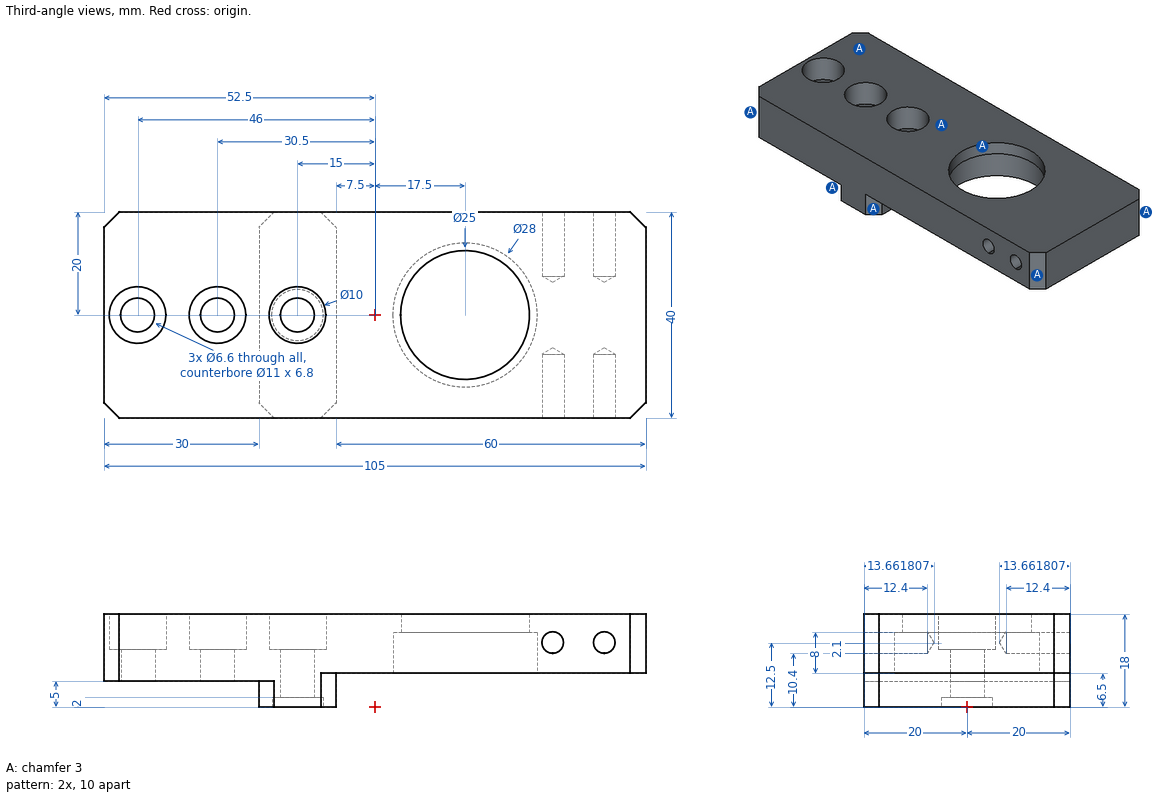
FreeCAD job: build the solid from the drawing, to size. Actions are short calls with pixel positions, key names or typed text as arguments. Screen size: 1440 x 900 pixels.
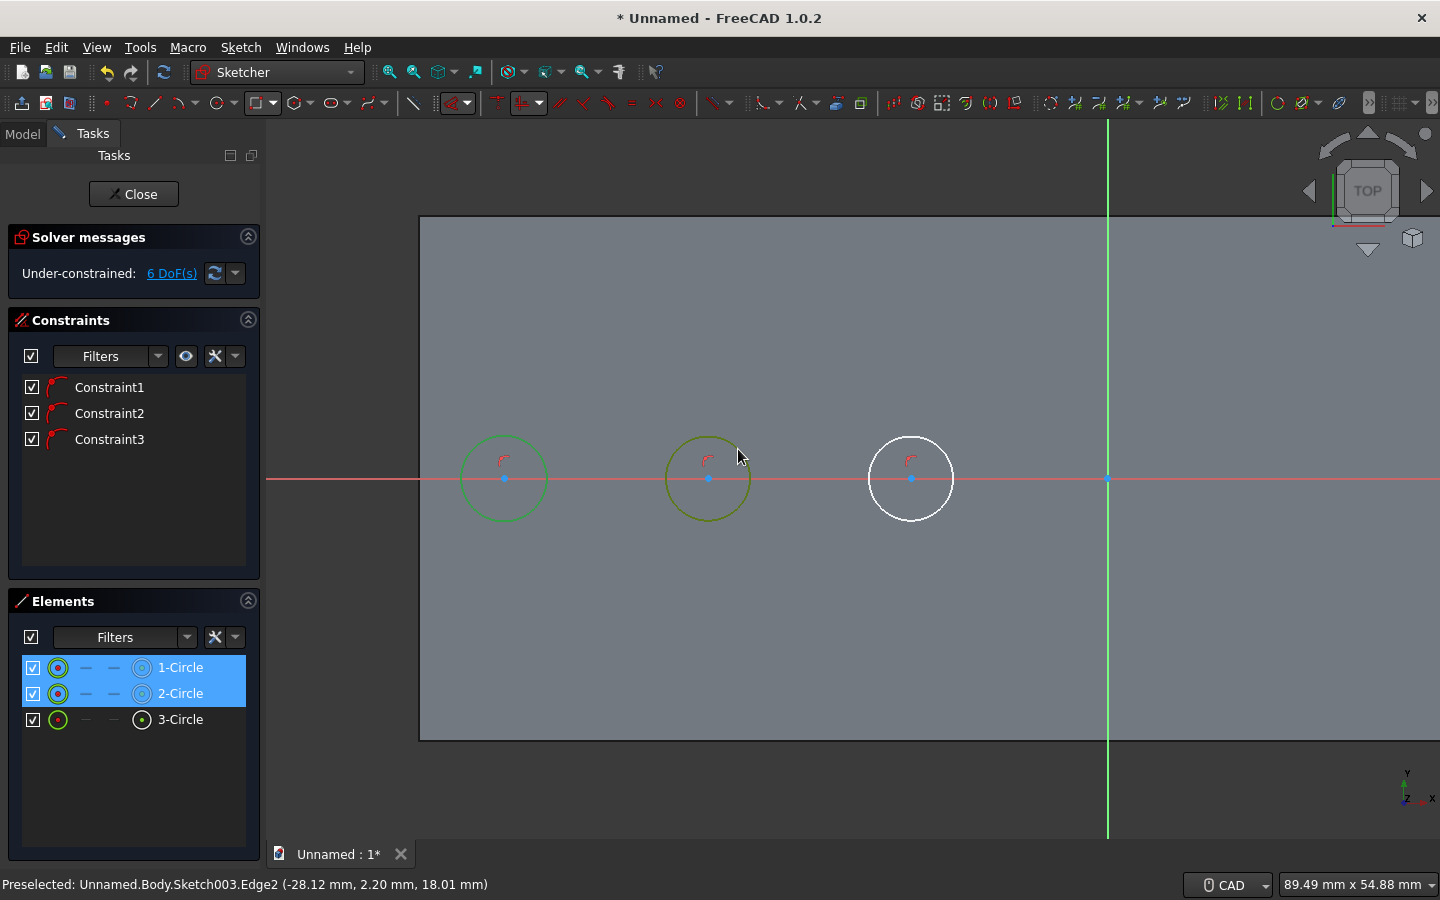
click(941, 449)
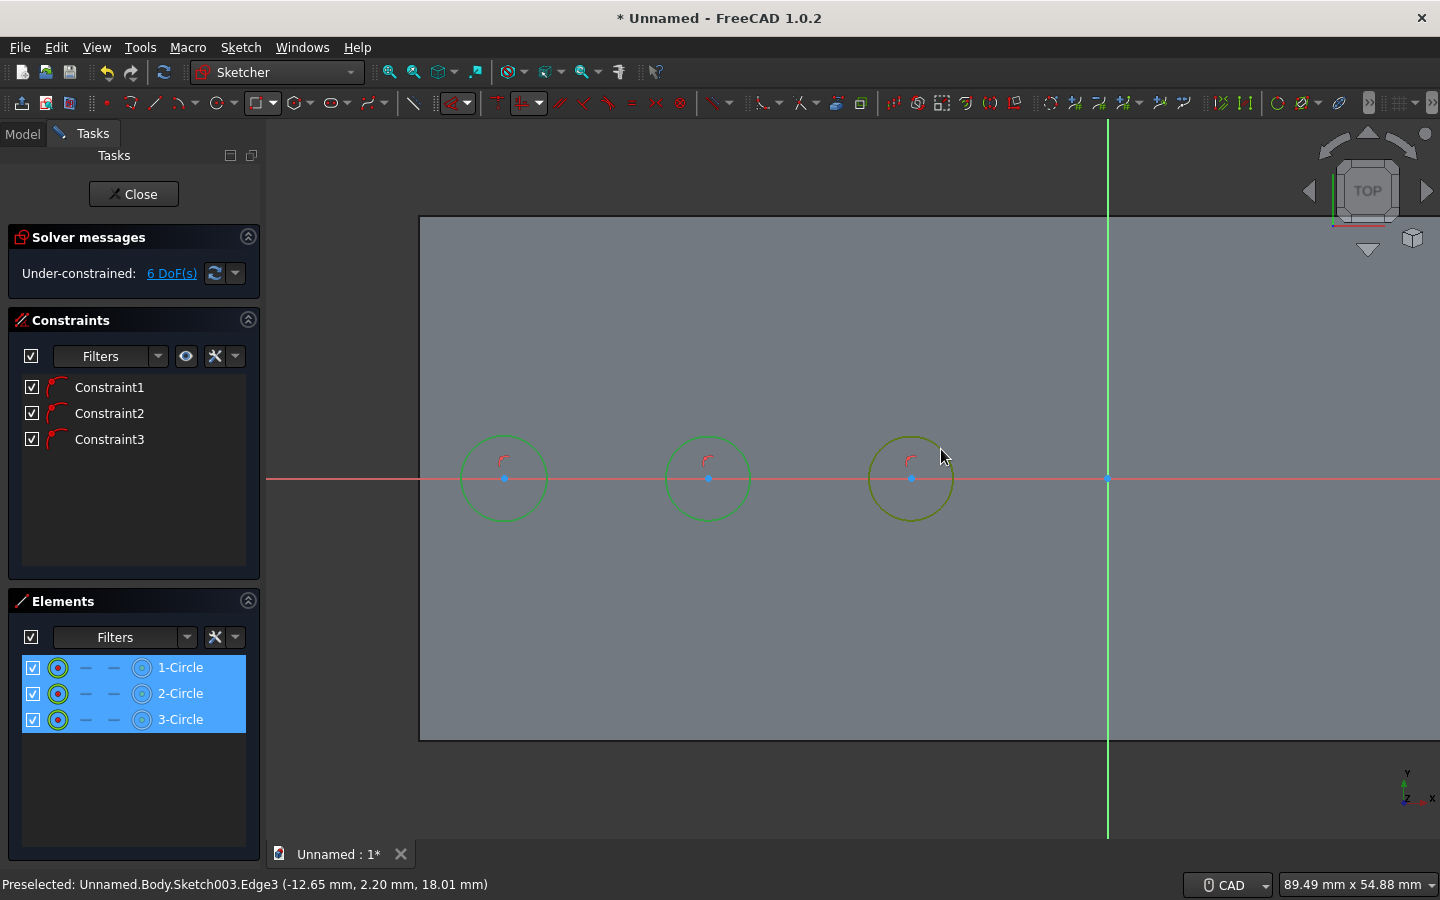
click(632, 104)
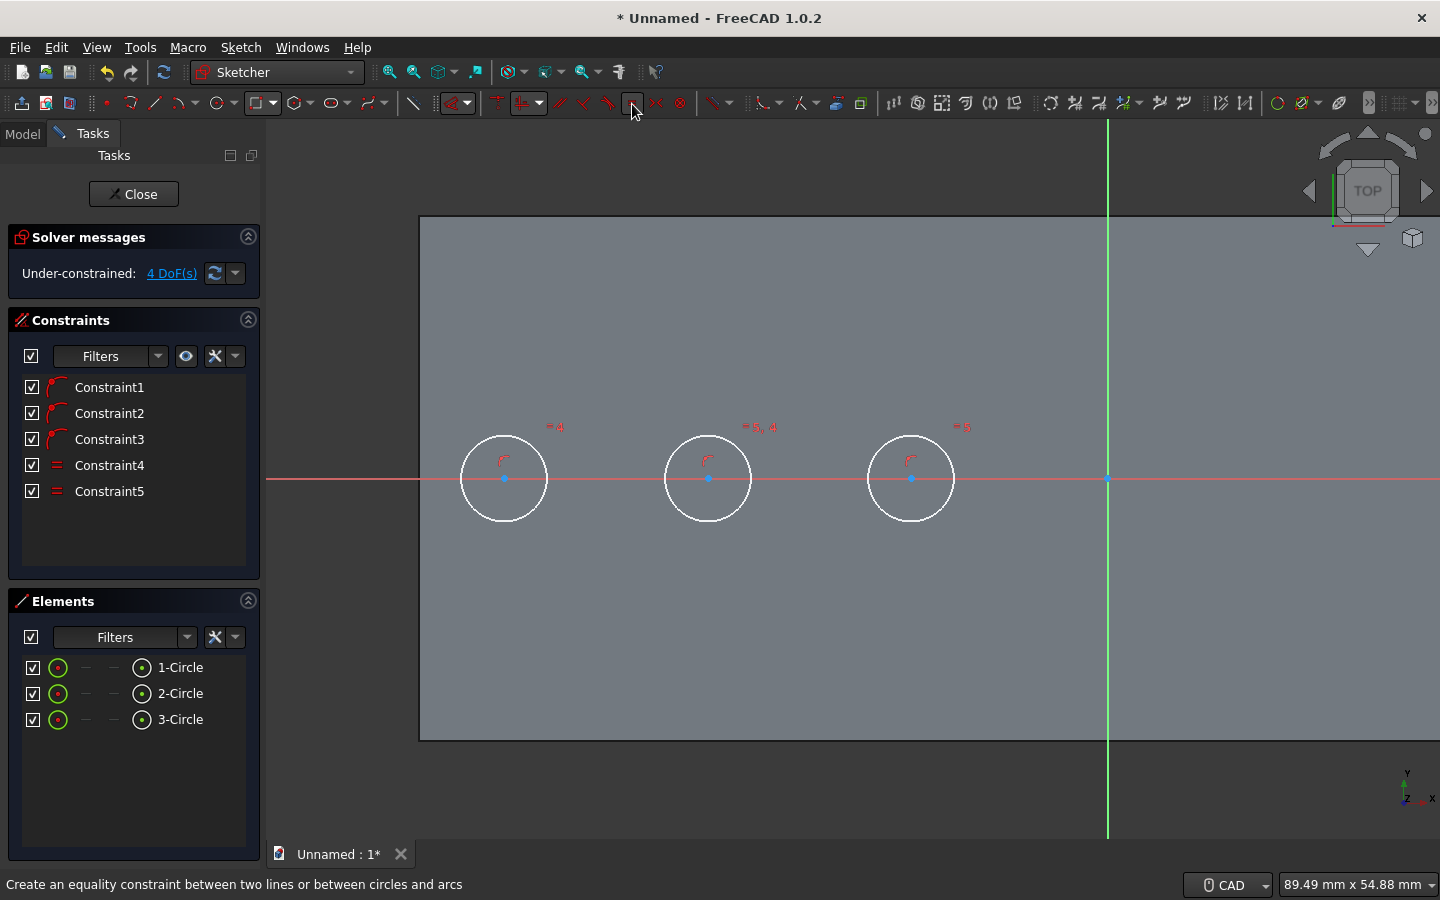
click(534, 448)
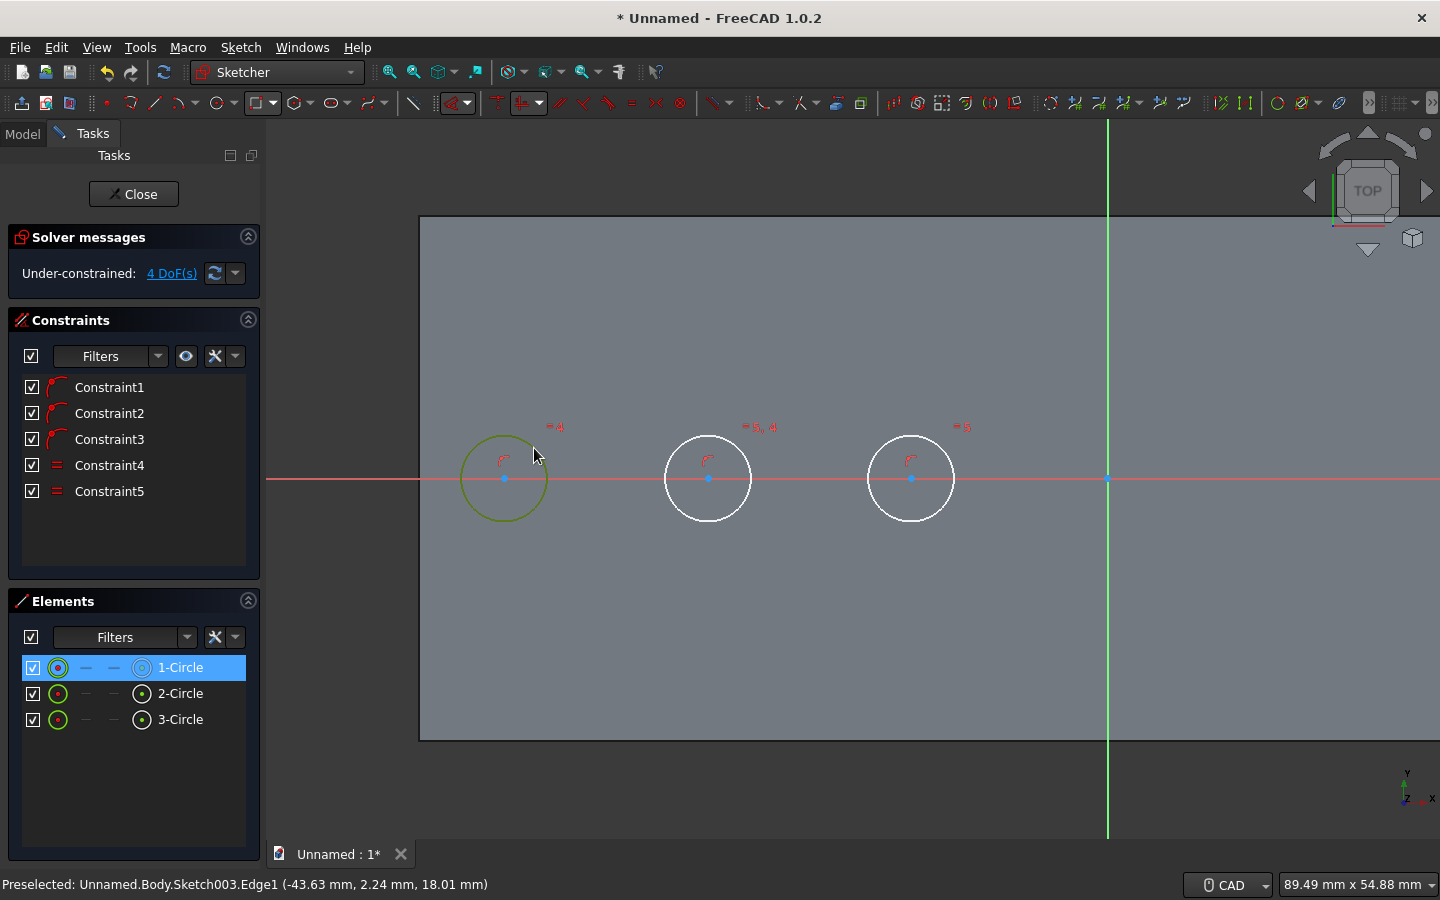
click(470, 104)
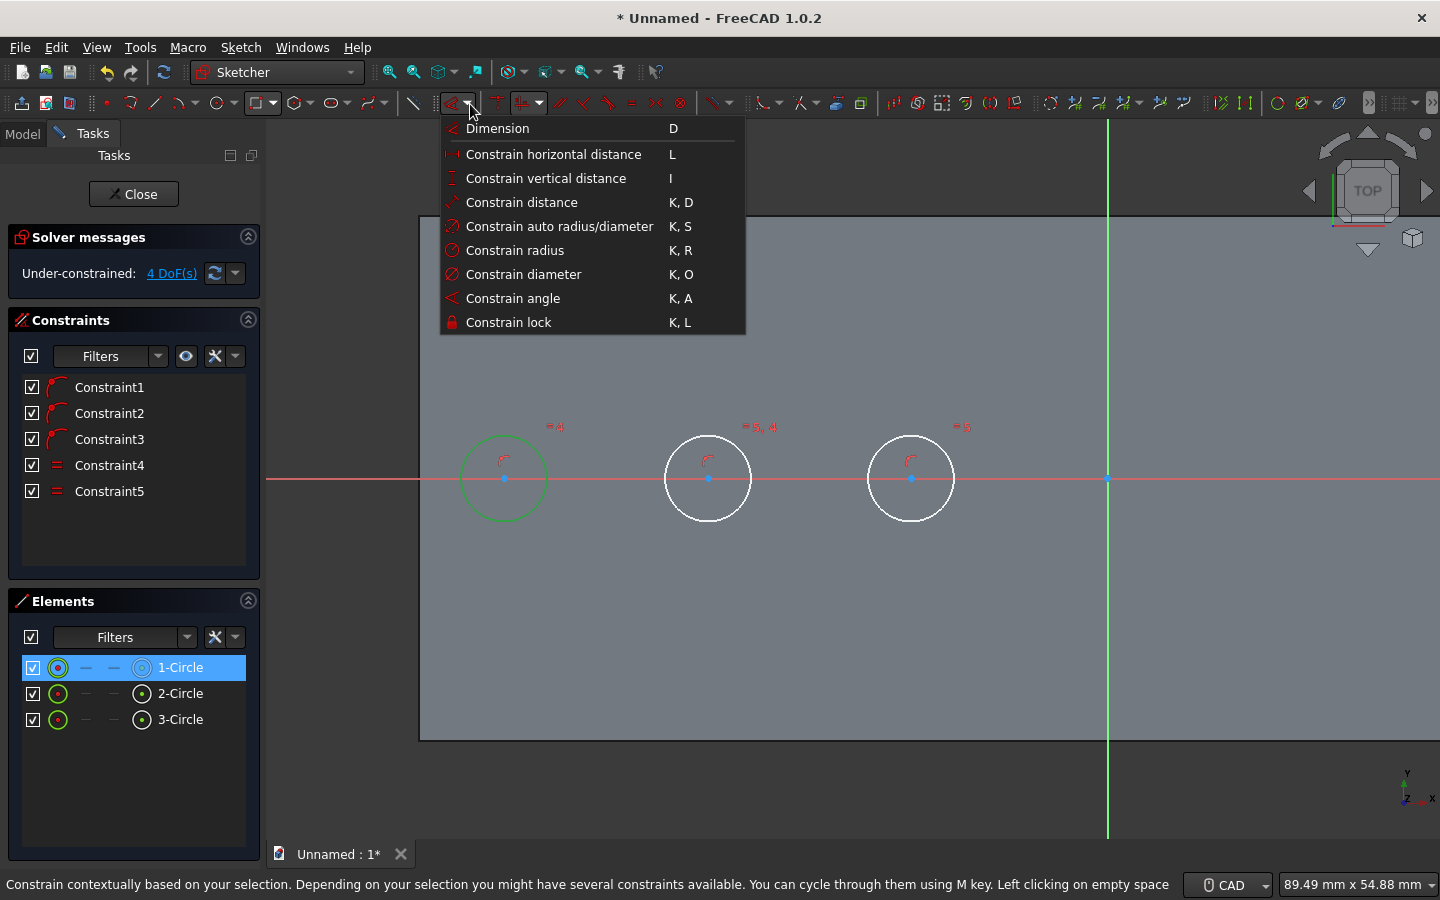
click(593, 274)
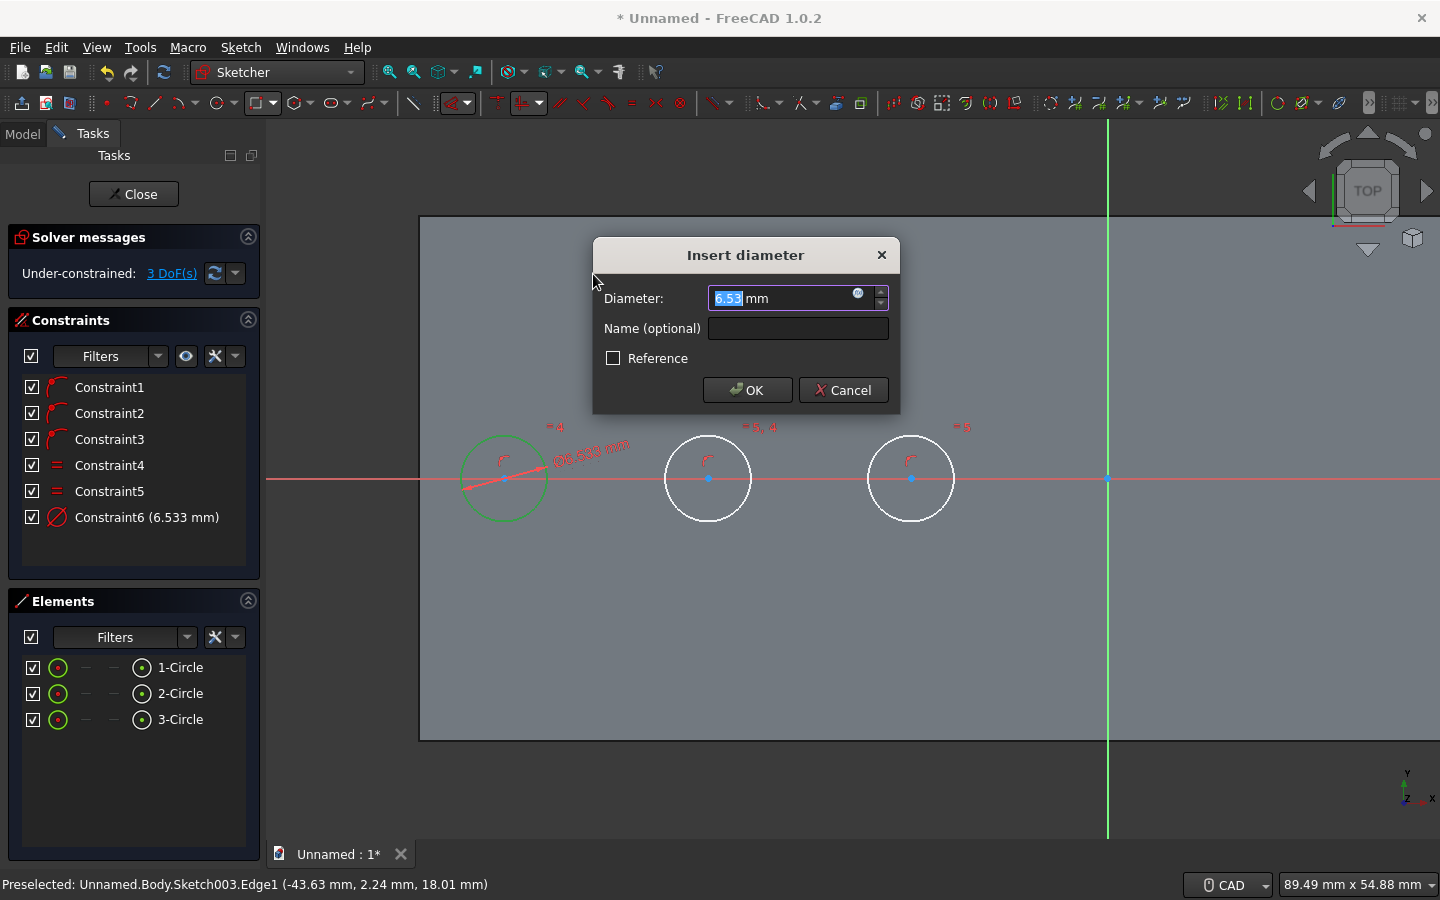
text(6.6)
key(Return)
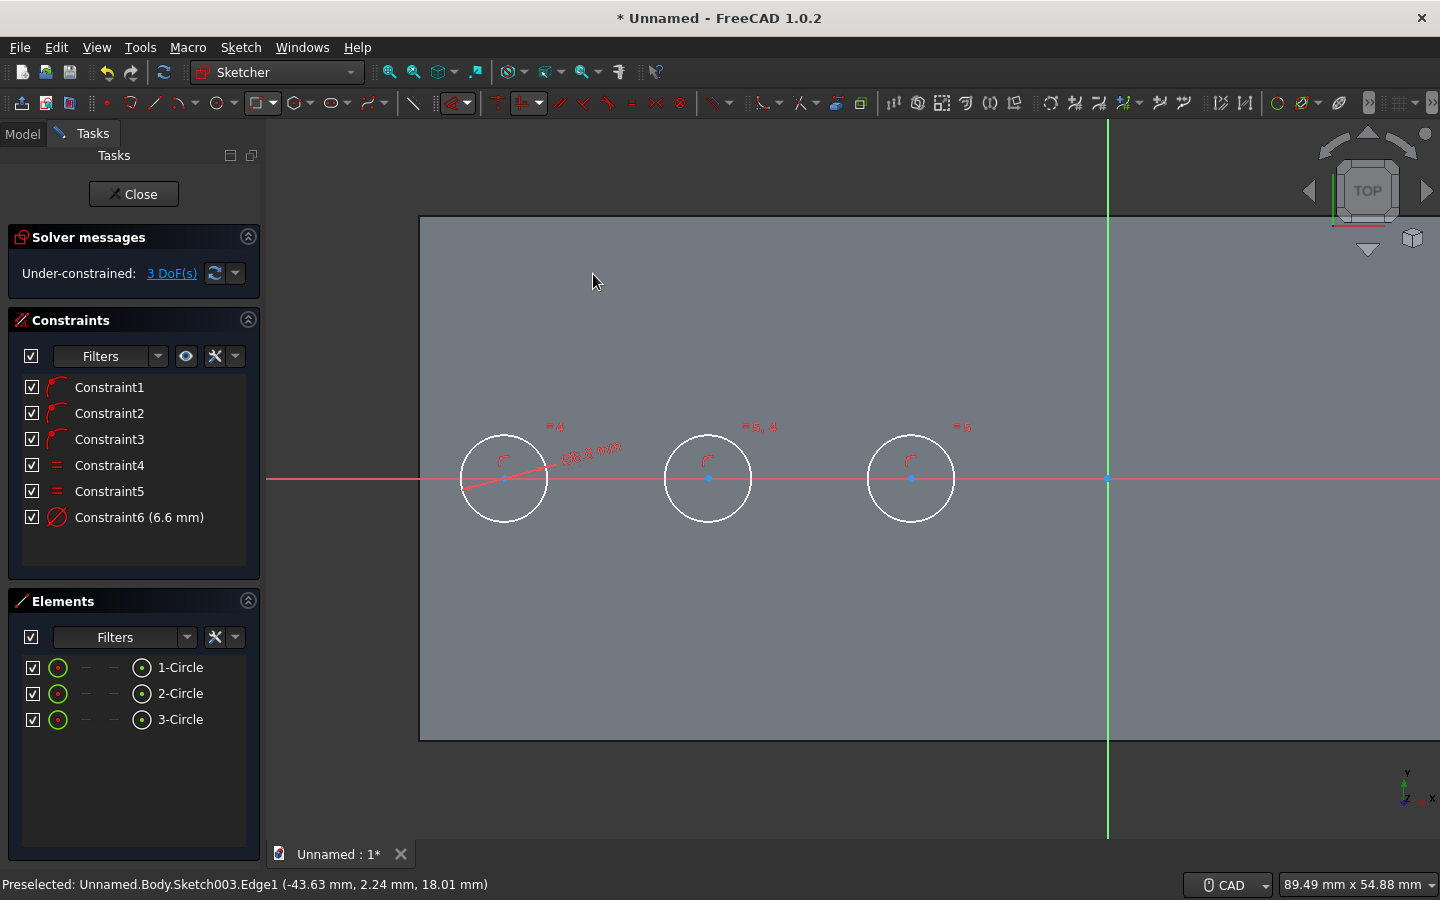
click(504, 479)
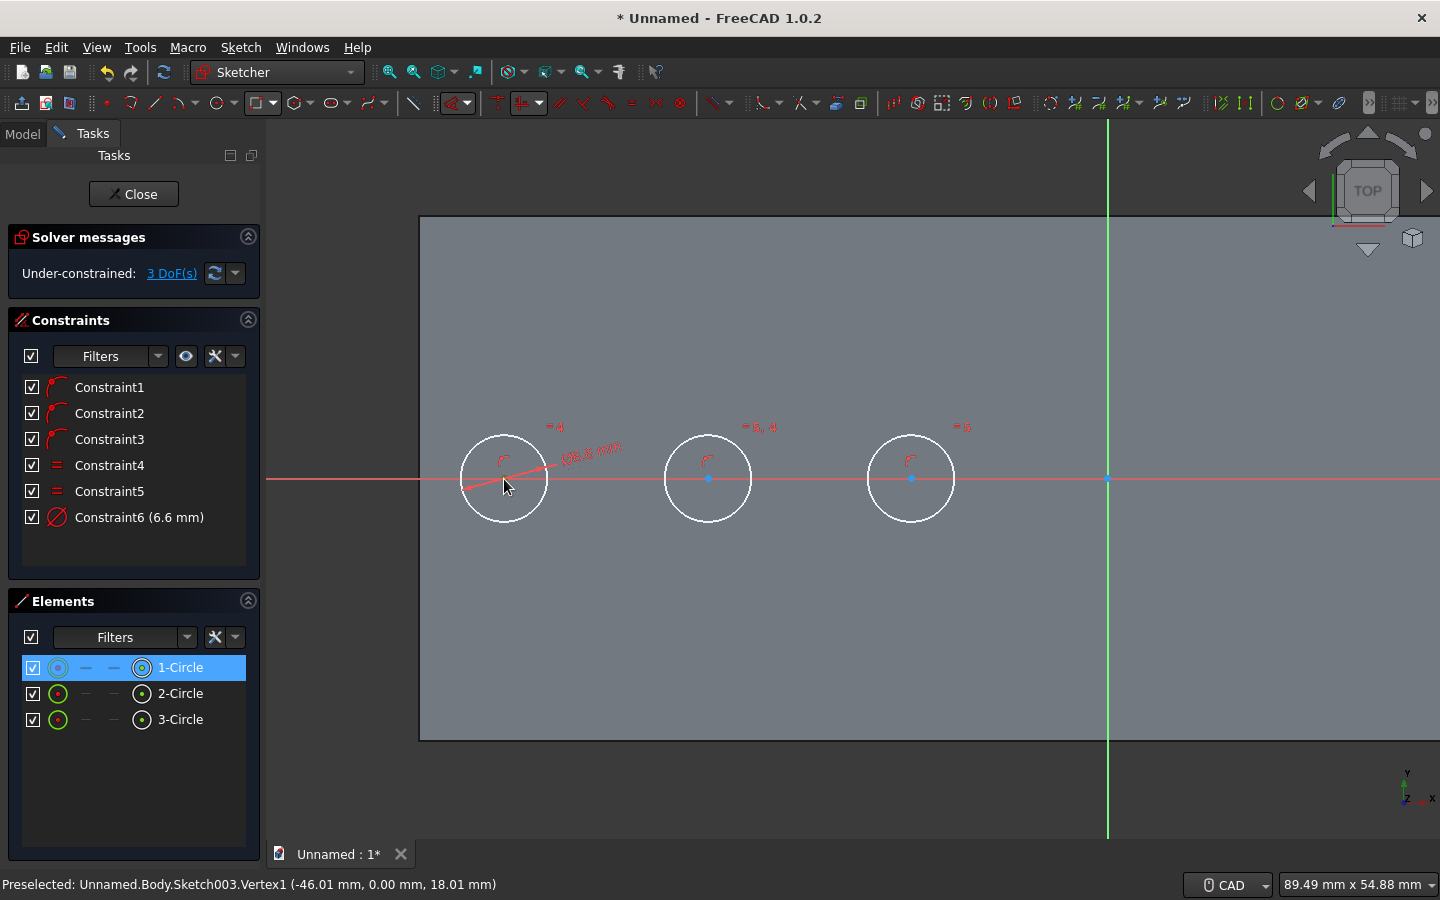
key(l)